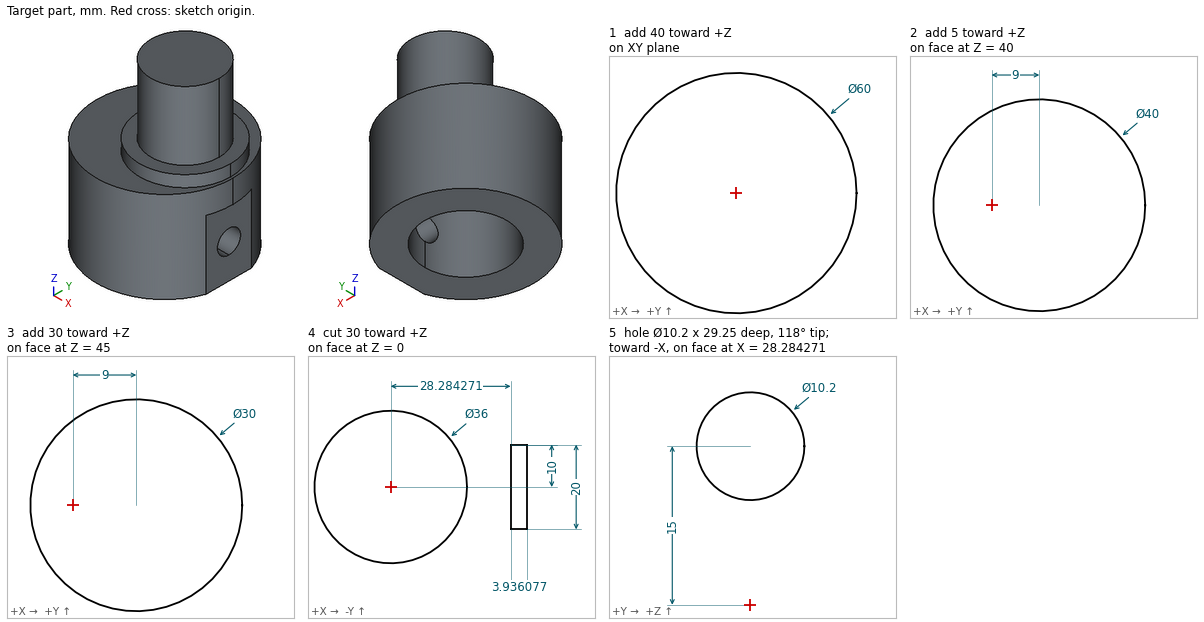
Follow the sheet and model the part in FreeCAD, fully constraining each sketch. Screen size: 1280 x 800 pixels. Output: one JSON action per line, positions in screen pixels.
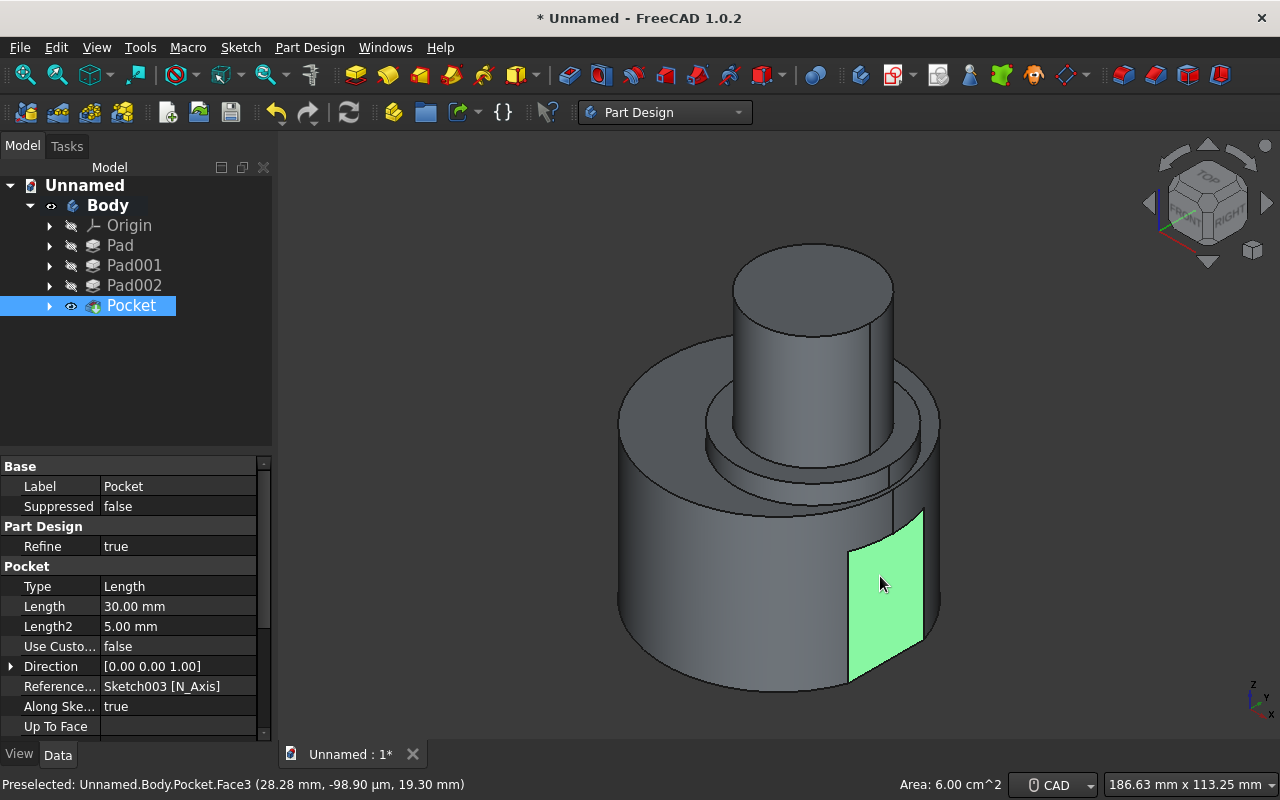
{"action": "left_click", "coordinate": [894, 76]}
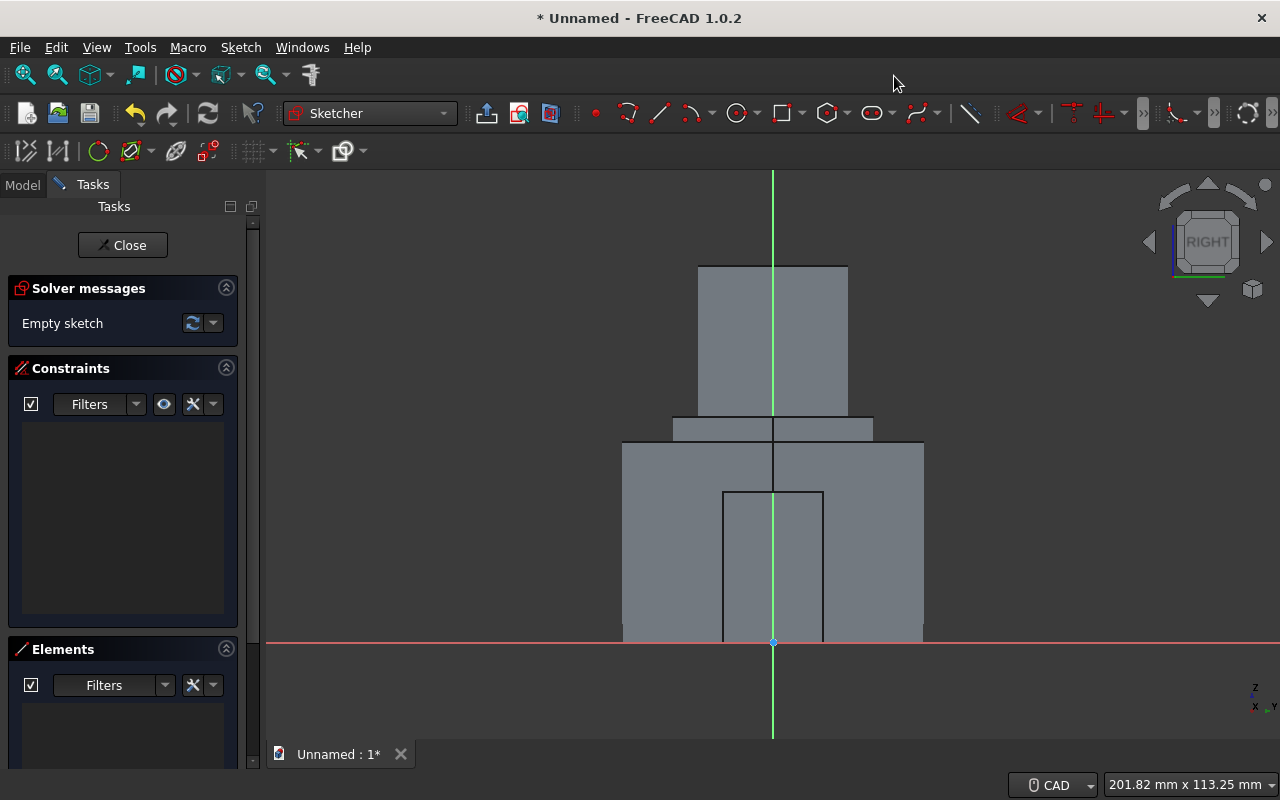
{"action": "scroll", "coordinate": [803, 652], "scroll_direction": "up", "scroll_amount": 6}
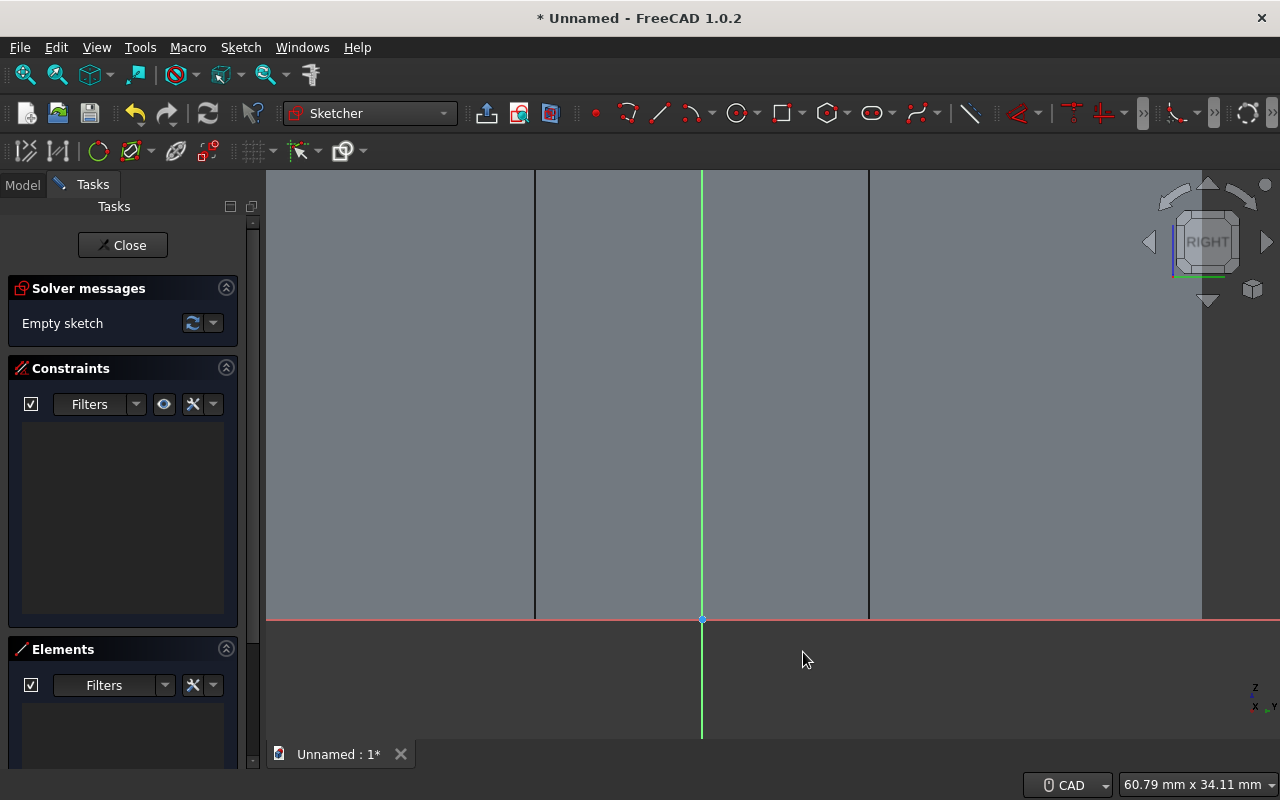
{"action": "key", "text": "g c"}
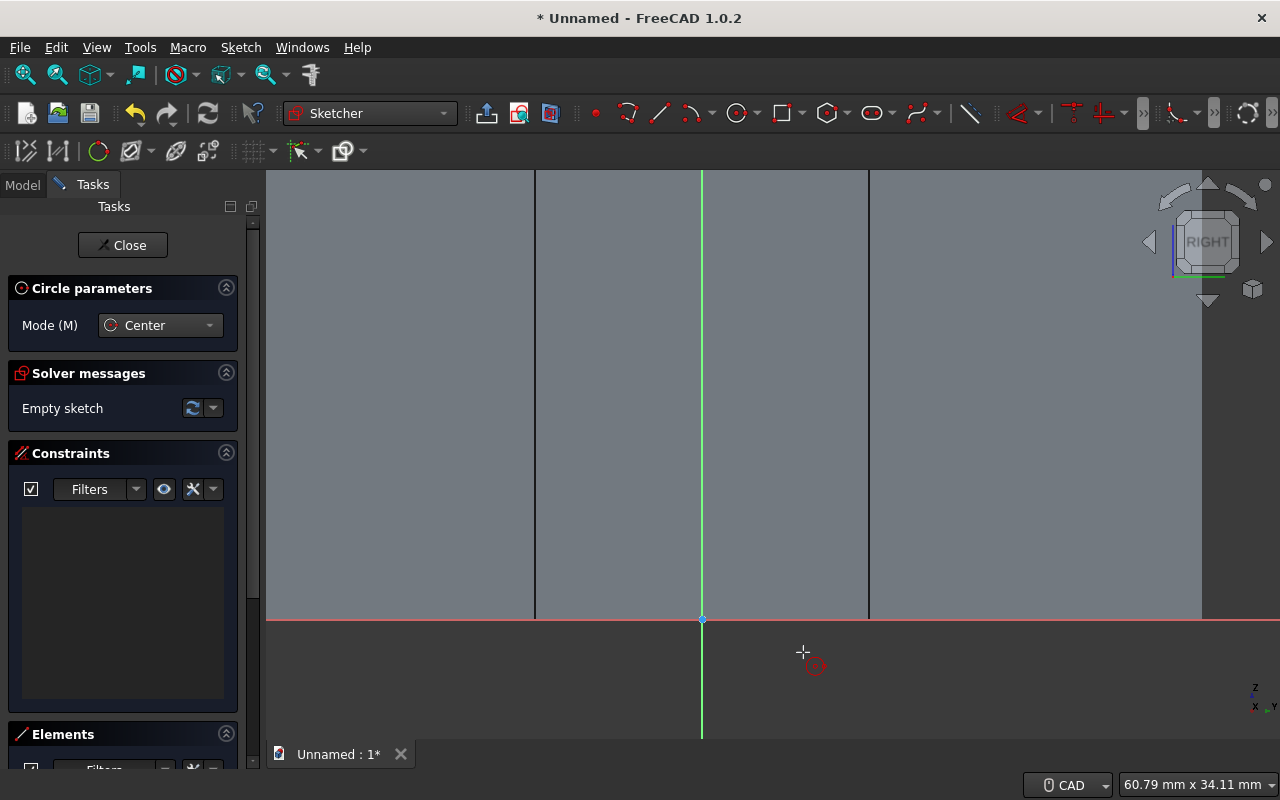
{"action": "left_click", "coordinate": [702, 370]}
{"action": "mouse_move", "coordinate": [762, 309]}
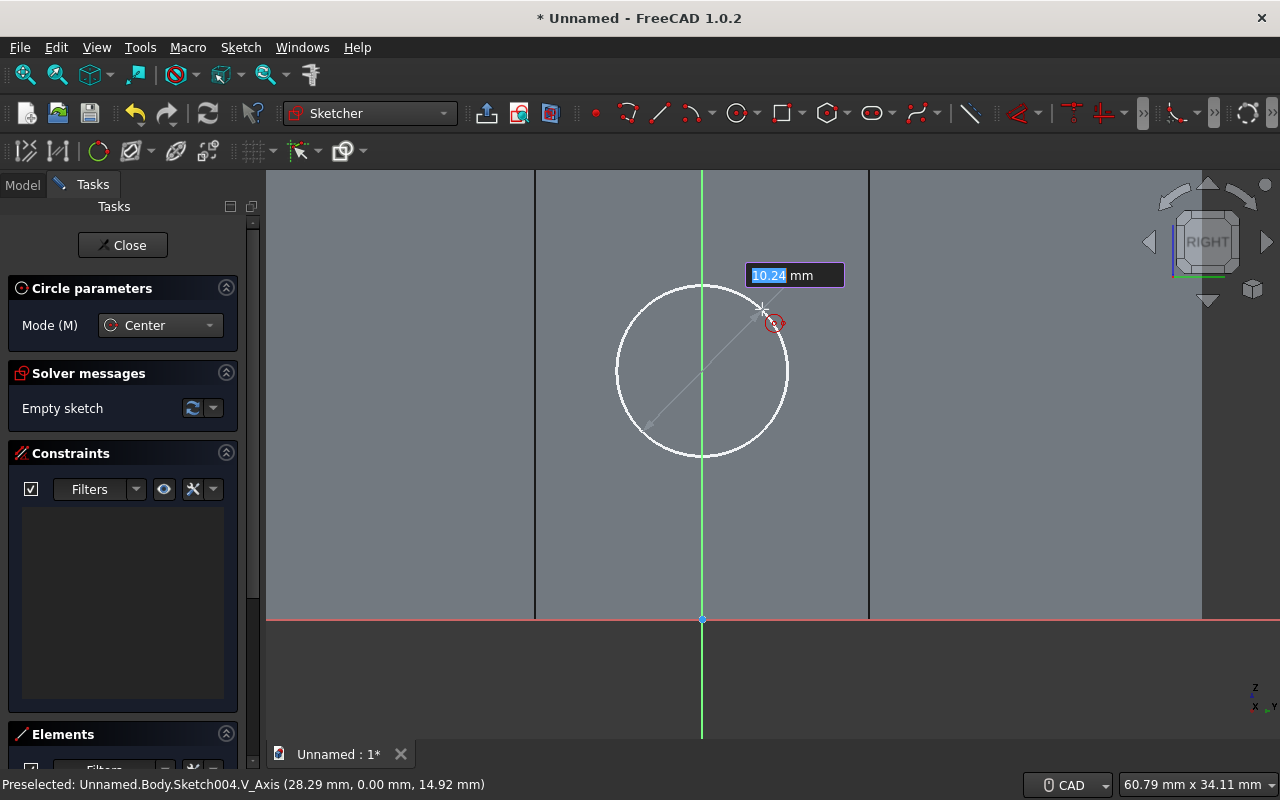
{"action": "type", "text": "10.2"}
{"action": "key", "text": "Return"}
{"action": "key", "text": "Escape"}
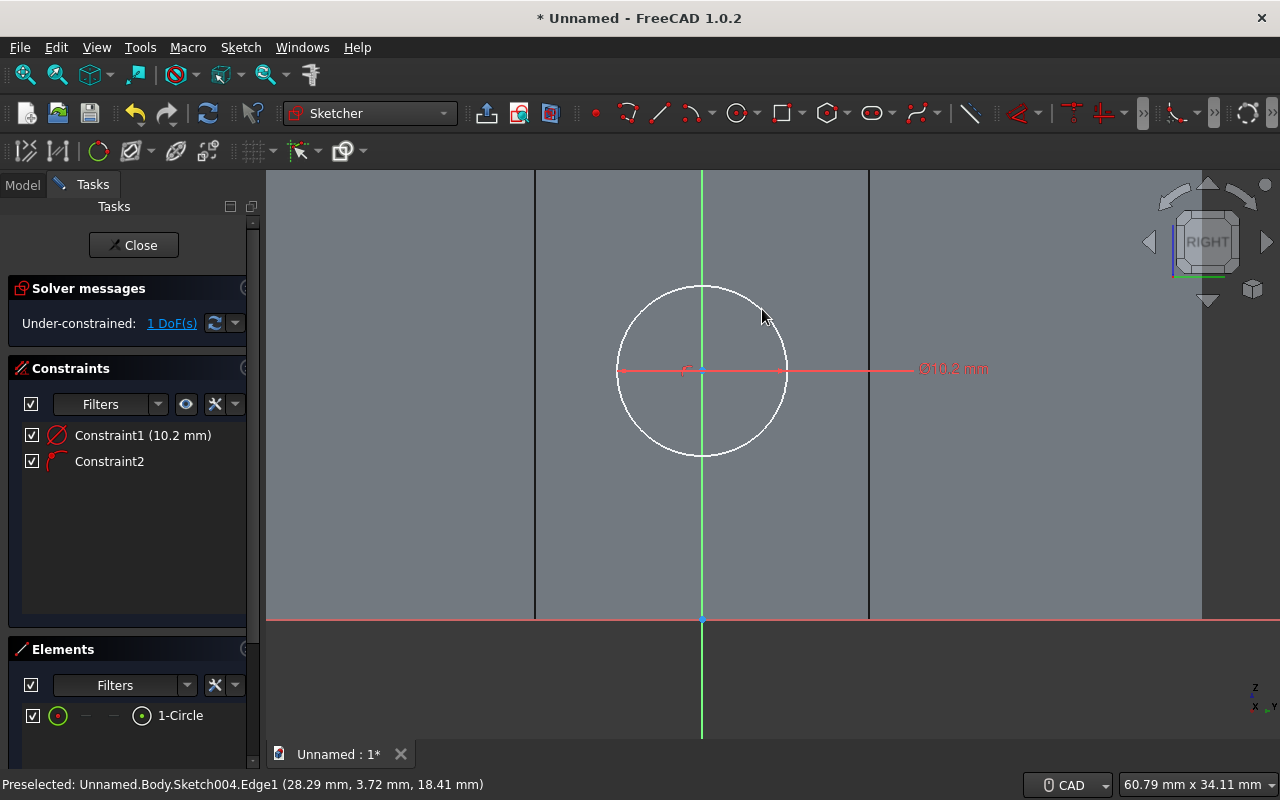
{"action": "left_click", "coordinate": [1018, 114]}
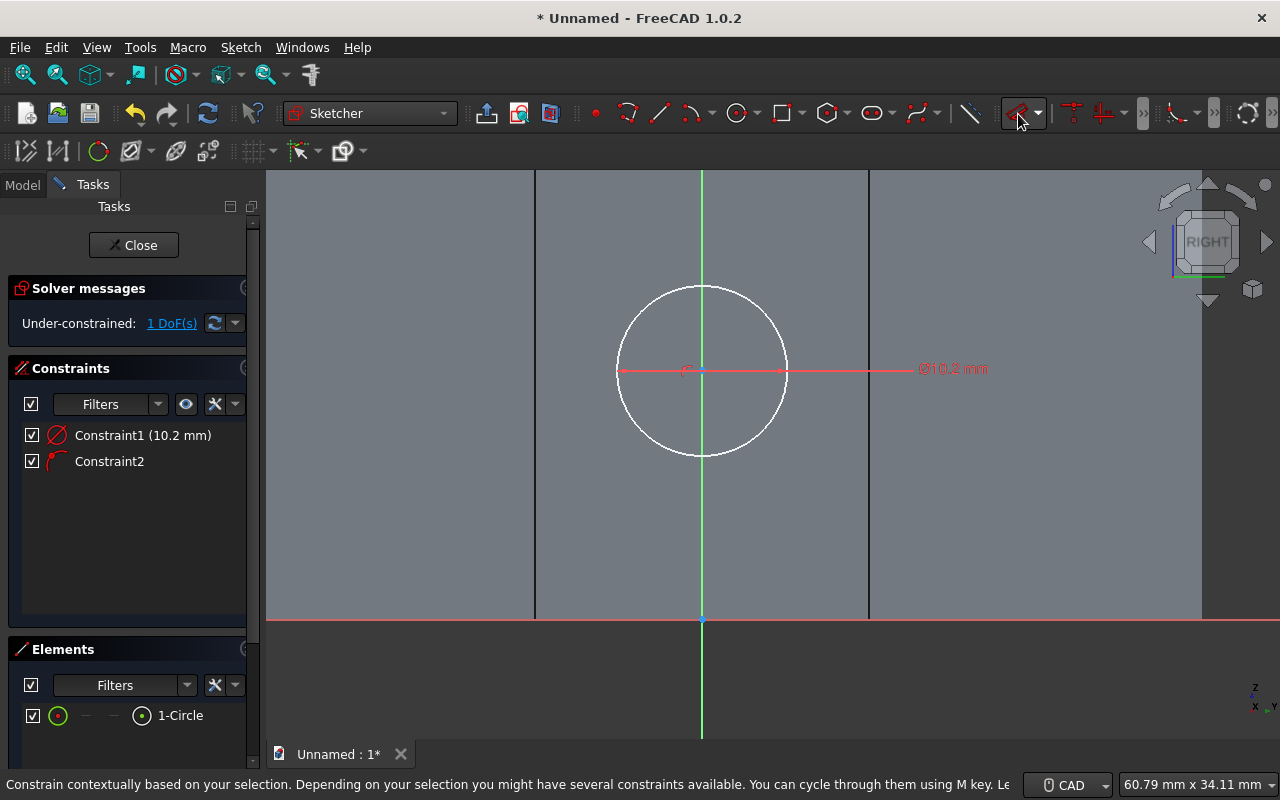
{"action": "left_click", "coordinate": [702, 371]}
{"action": "left_click", "coordinate": [736, 495]}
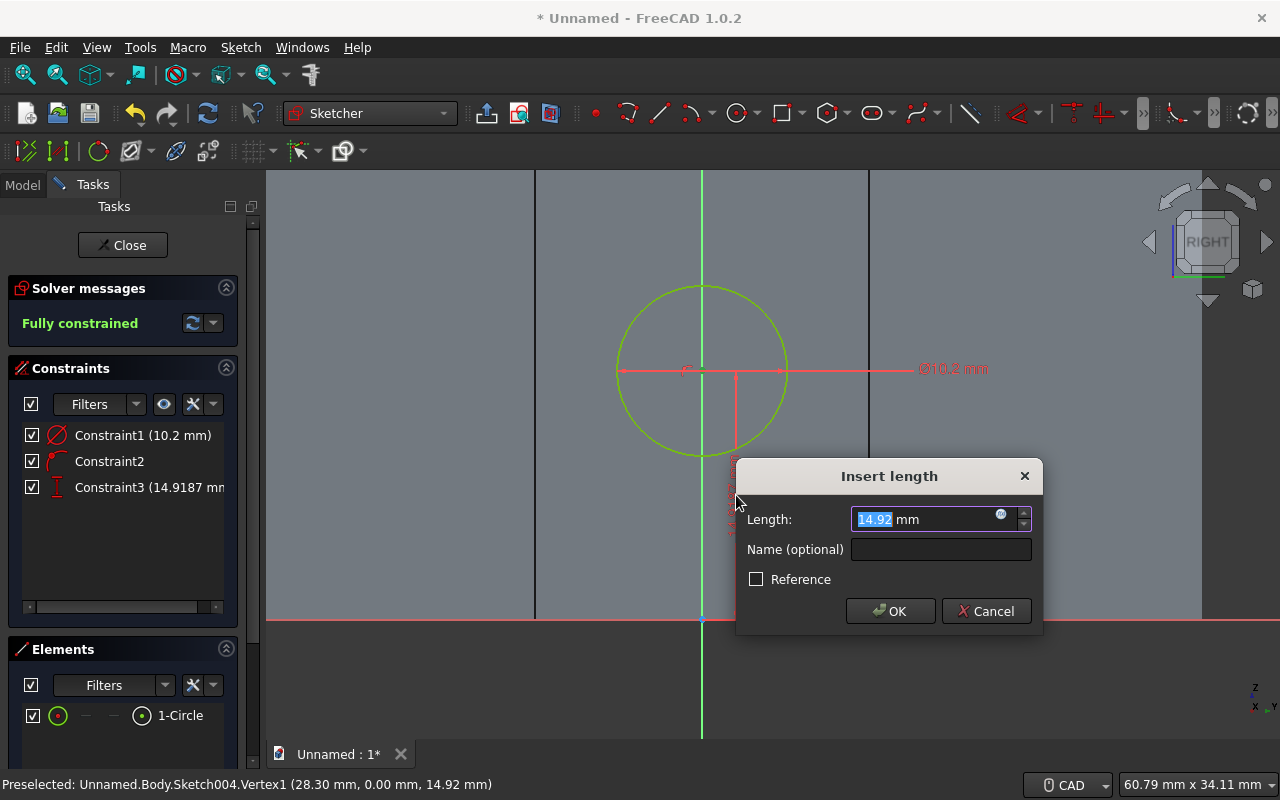
{"action": "type", "text": "15"}
{"action": "key", "text": "Return"}
{"action": "key", "text": "Escape"}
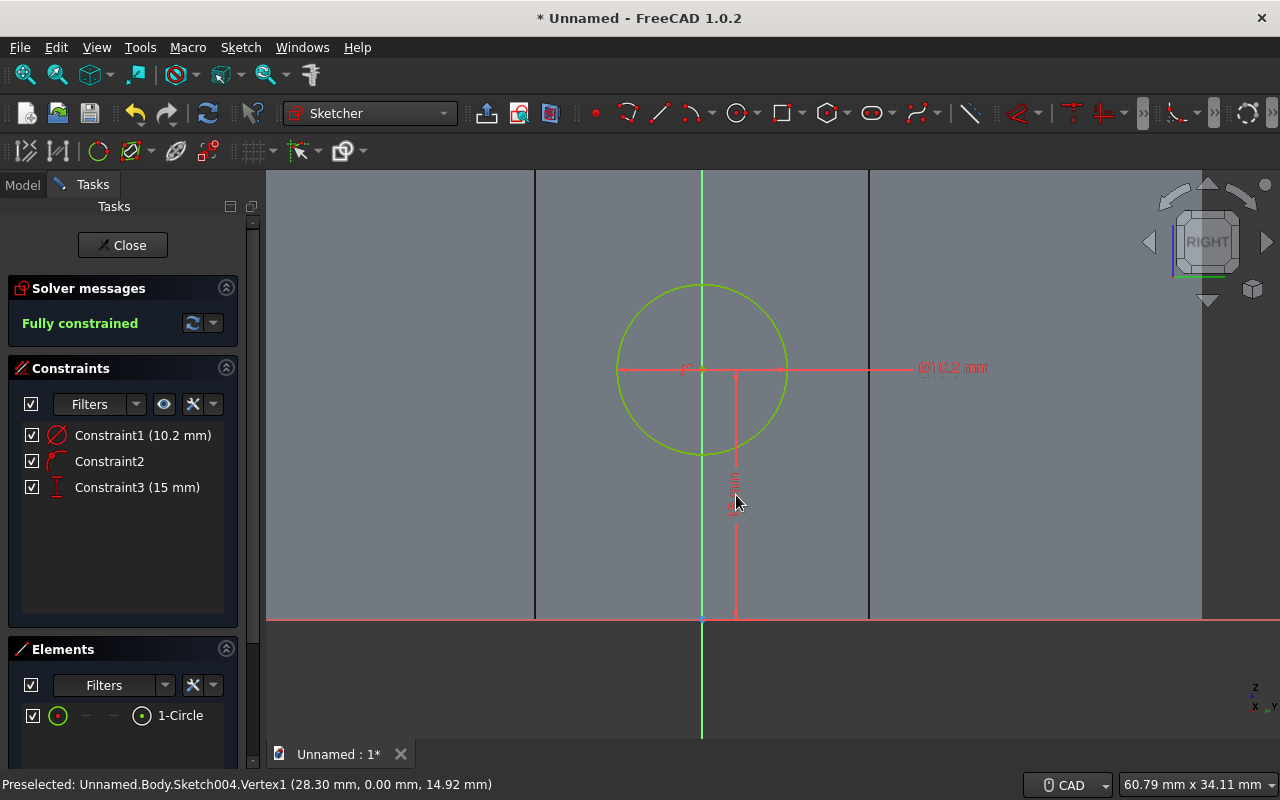
{"action": "left_click", "coordinate": [123, 245]}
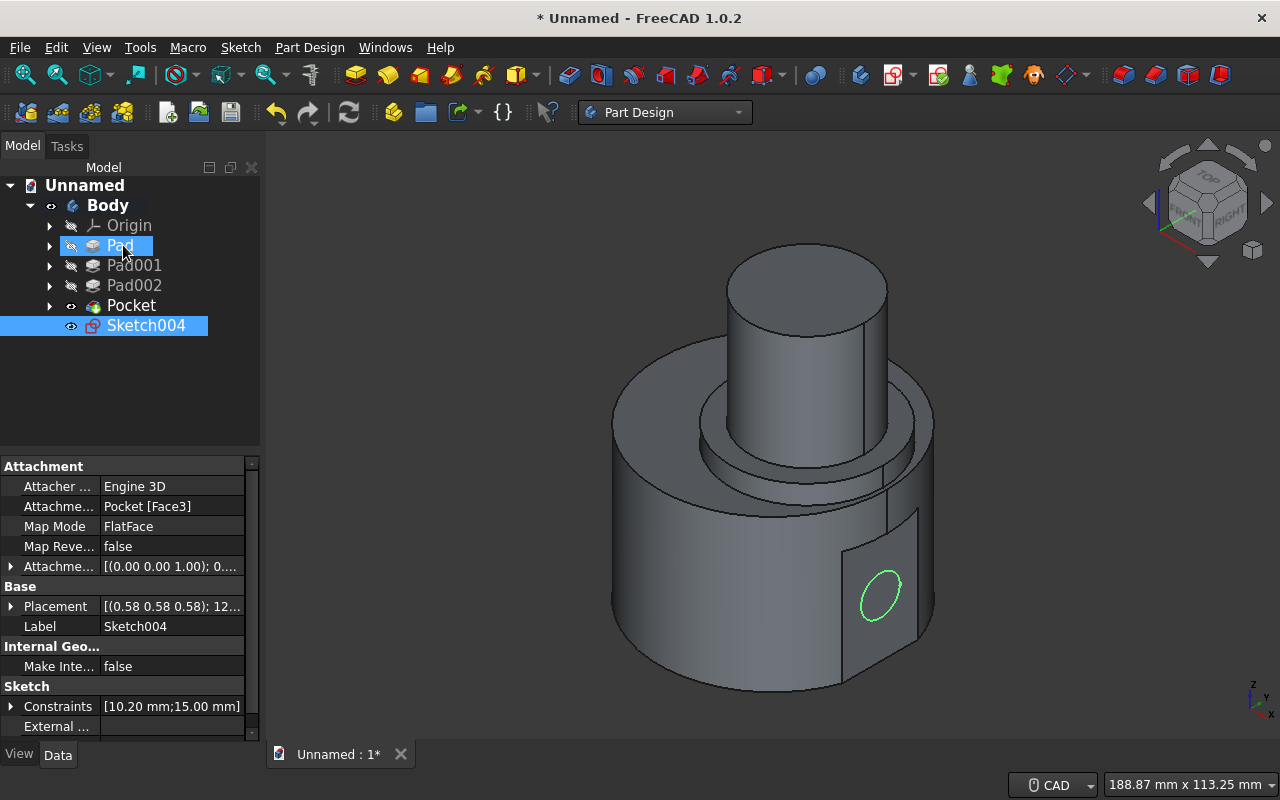
{"action": "left_click", "coordinate": [602, 76]}